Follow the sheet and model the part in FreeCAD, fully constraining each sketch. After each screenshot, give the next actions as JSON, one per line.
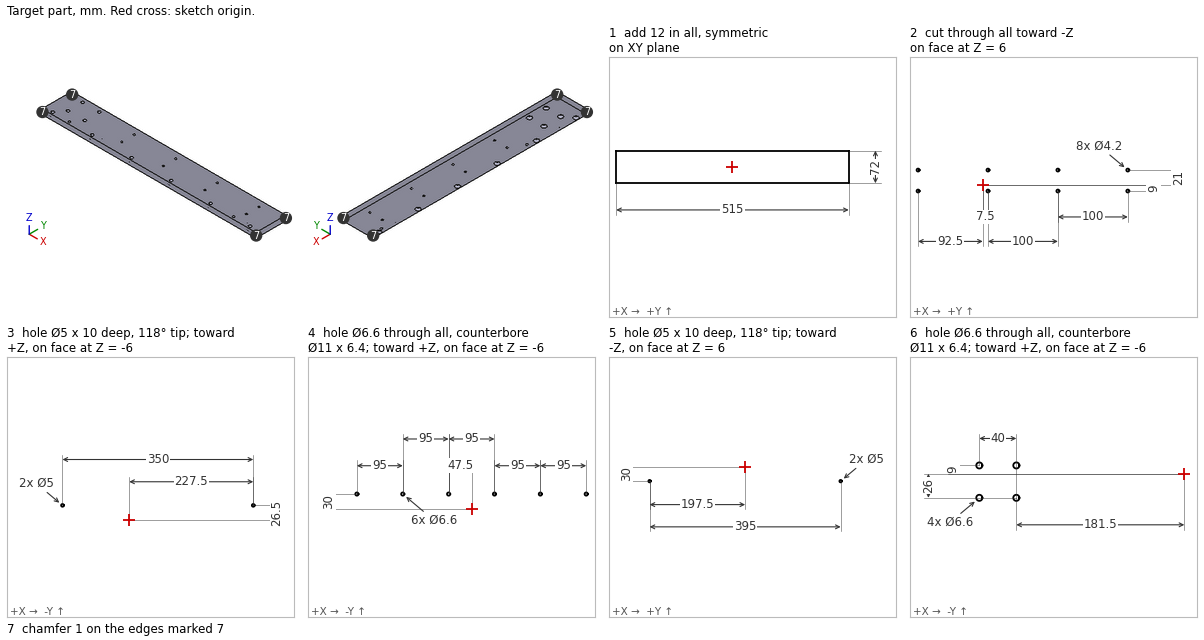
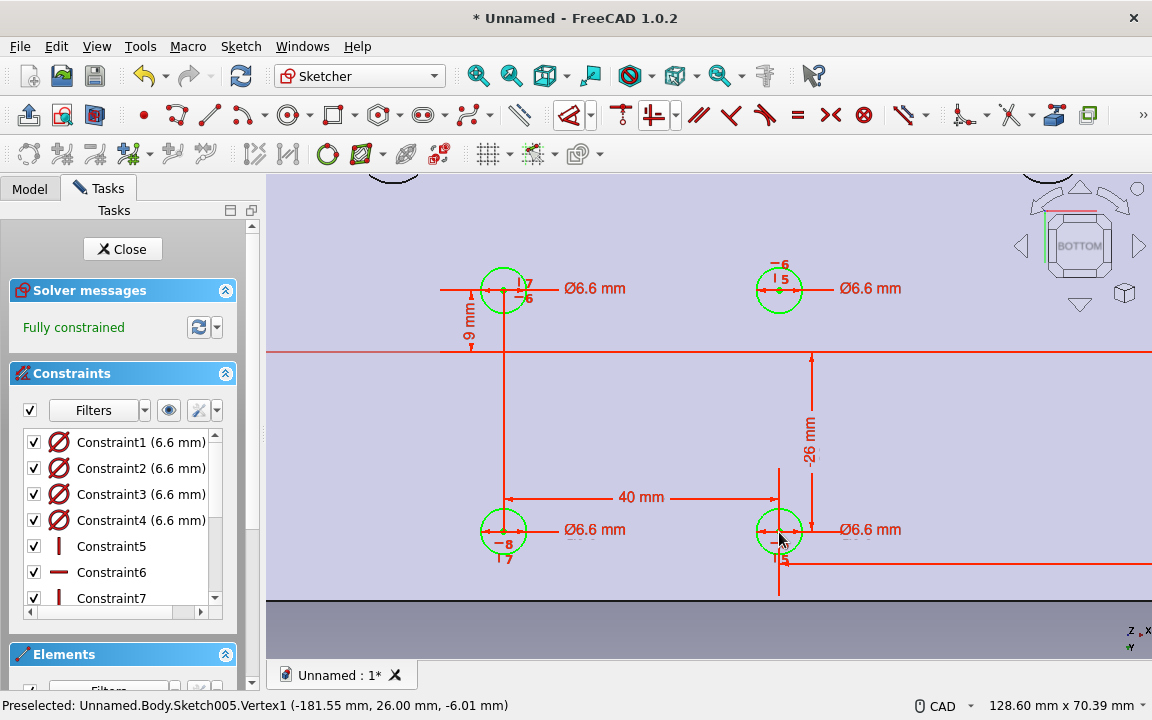
{"action": "left_click", "coordinate": [123, 249]}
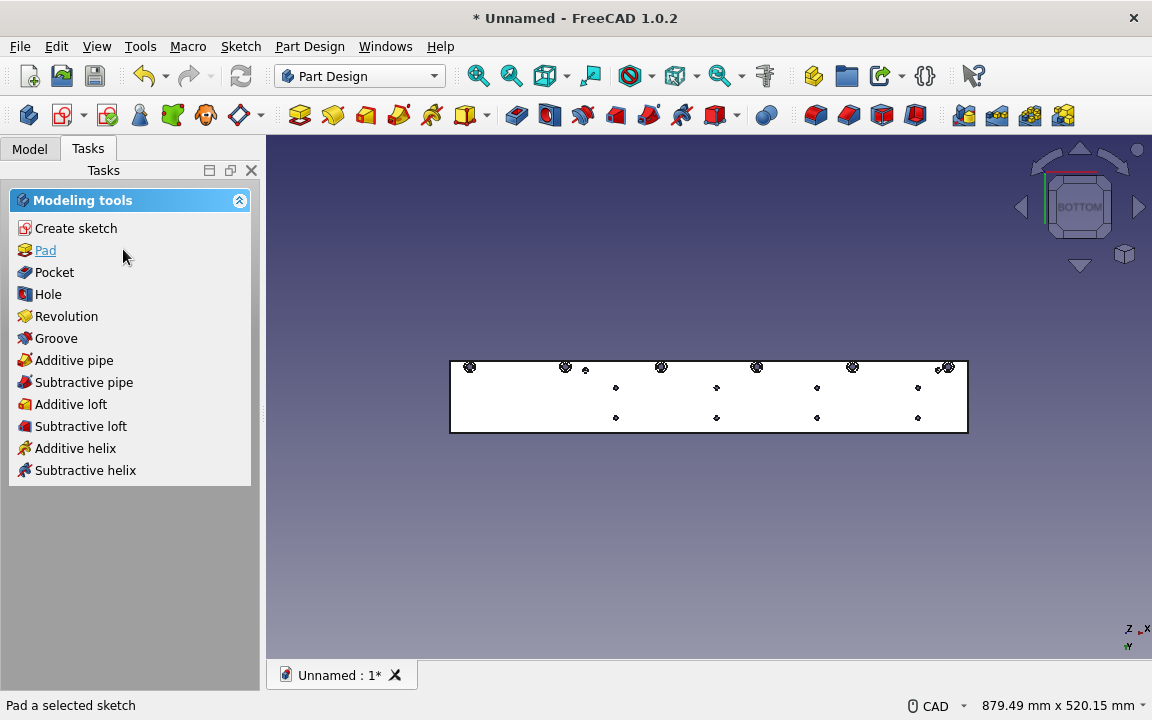
{"action": "left_click", "coordinate": [550, 116]}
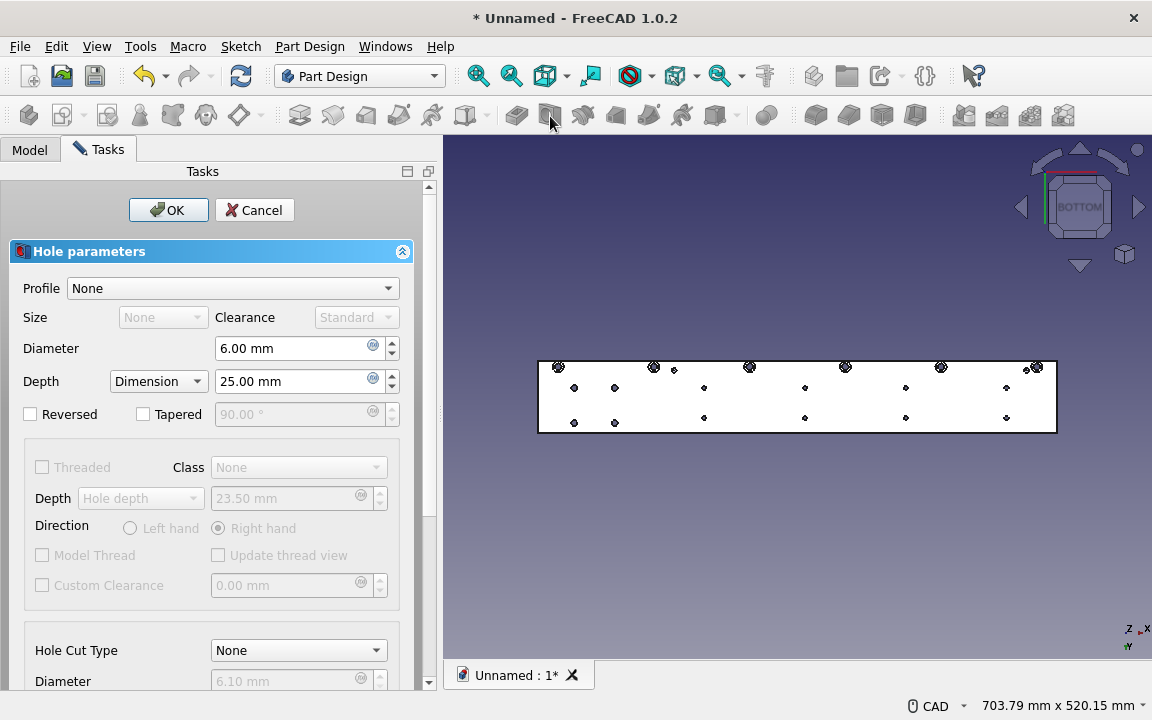
{"action": "triple_click", "coordinate": [300, 348]}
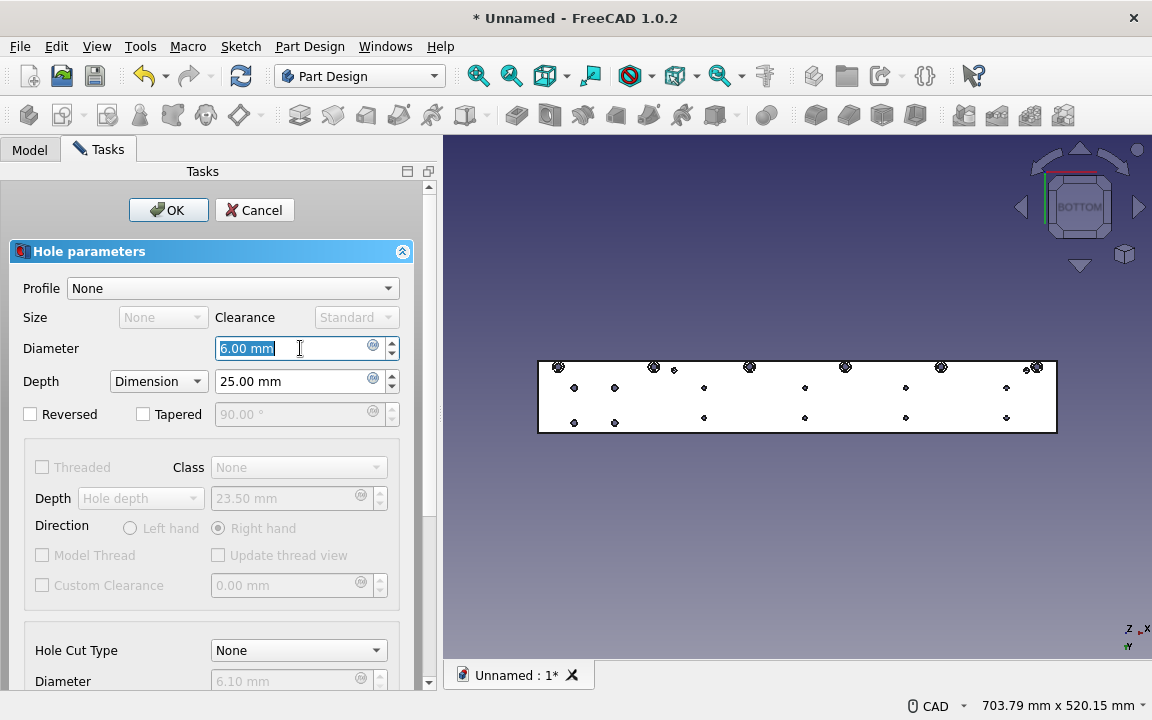
{"action": "type", "text": "6.6"}
{"action": "key", "text": "Tab"}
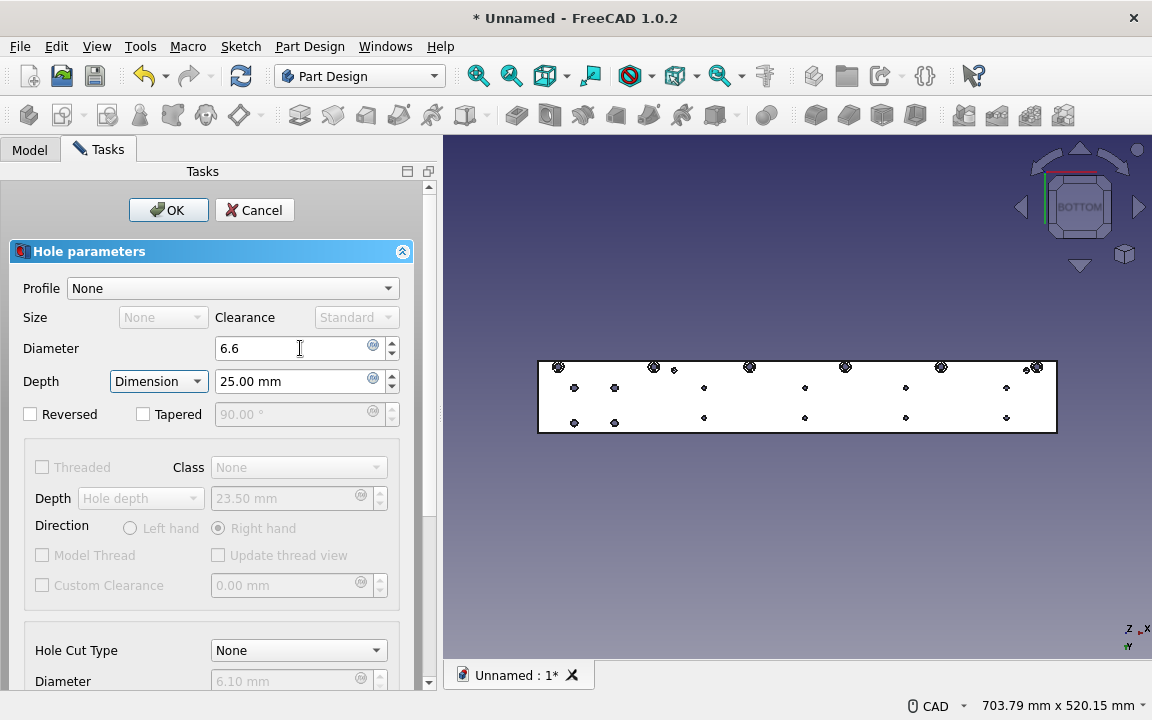
{"action": "left_click", "coordinate": [160, 382]}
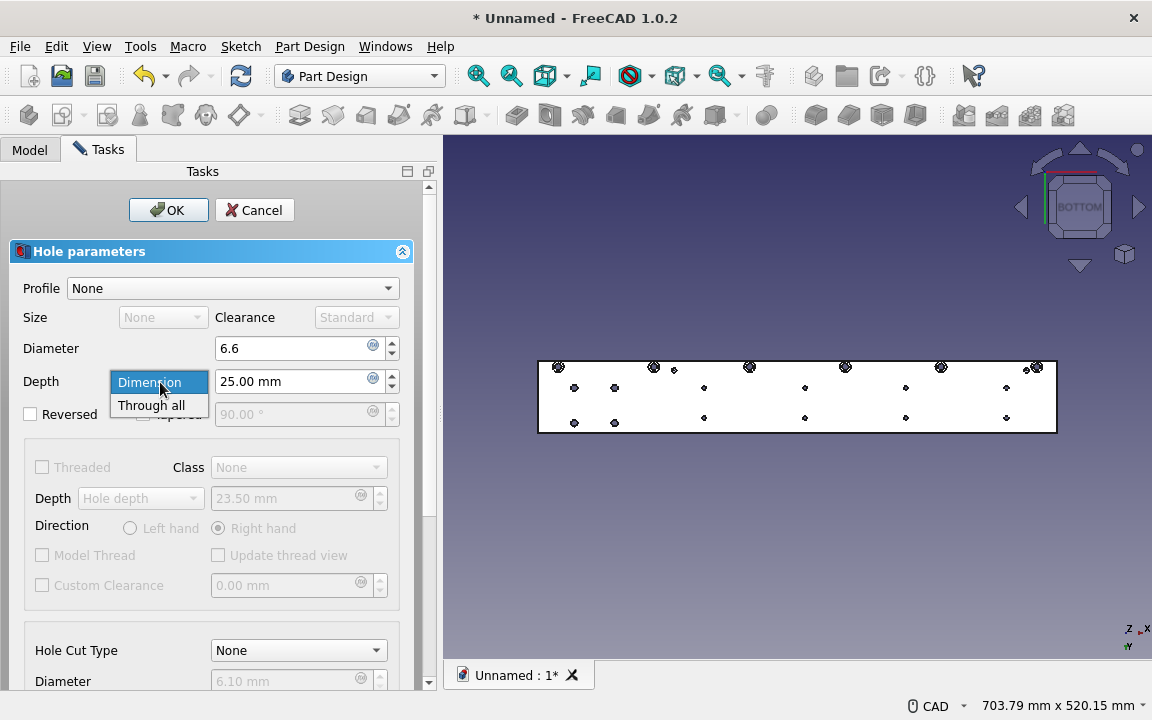
{"action": "left_click", "coordinate": [158, 406]}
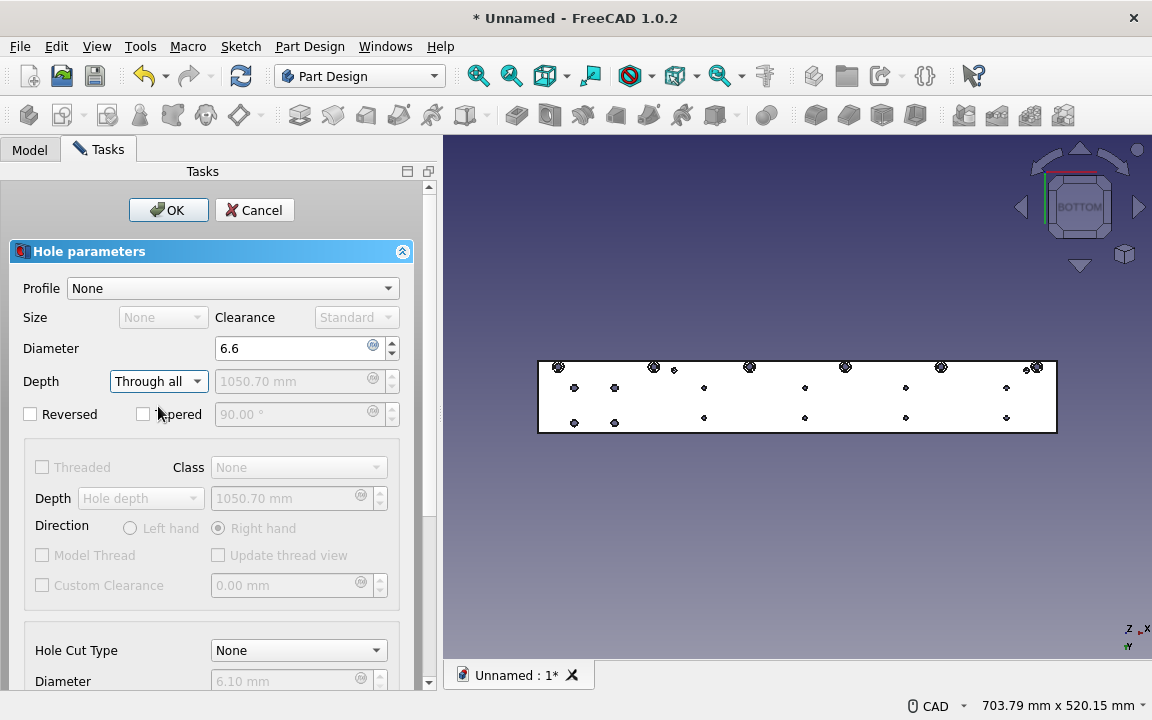
{"action": "left_click", "coordinate": [300, 650]}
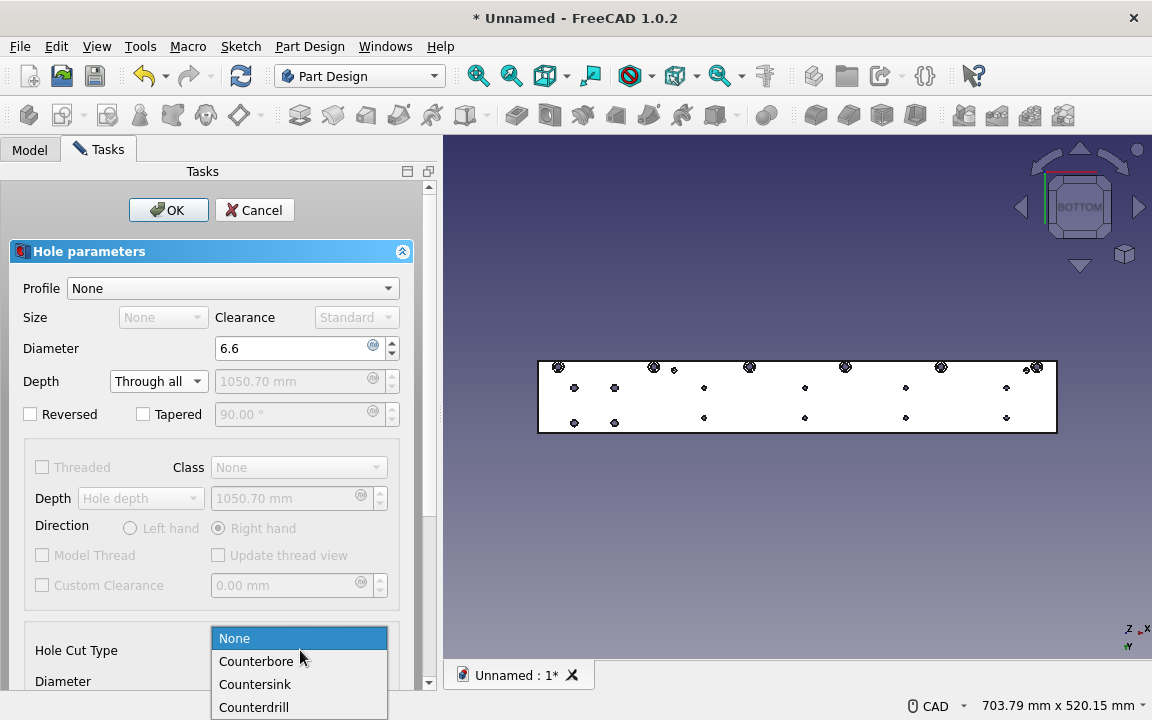
{"action": "left_click", "coordinate": [298, 662]}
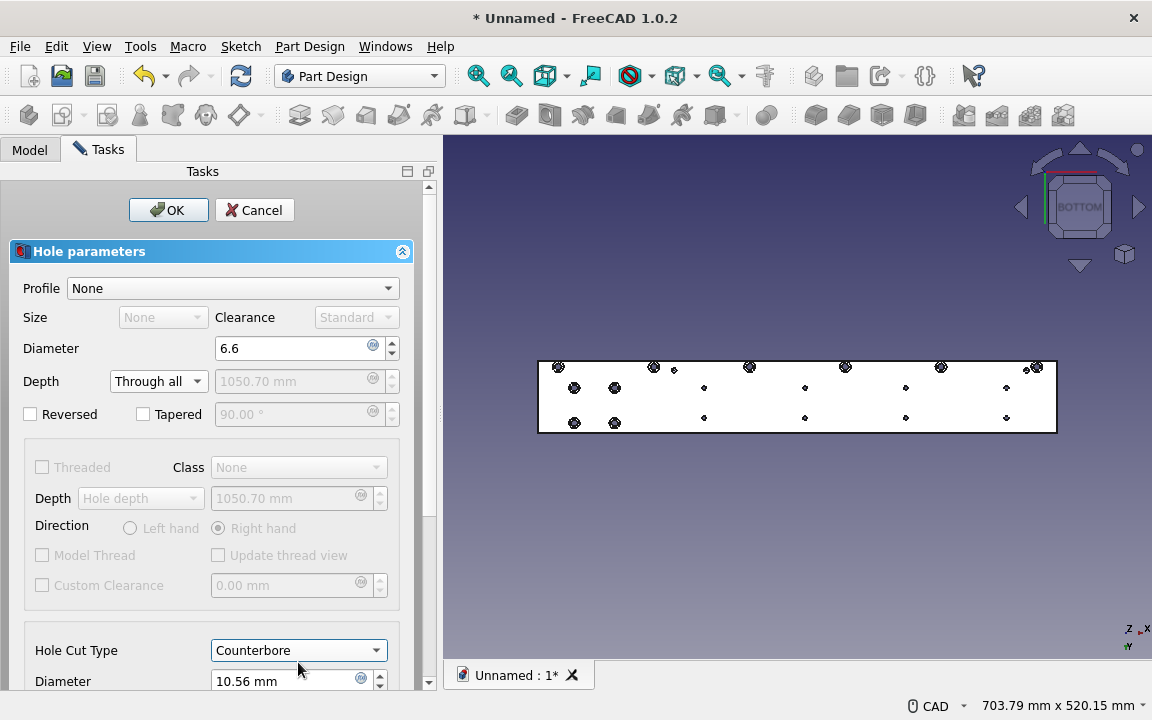
{"action": "scroll", "coordinate": [429, 436], "scroll_direction": "down", "scroll_amount": 2}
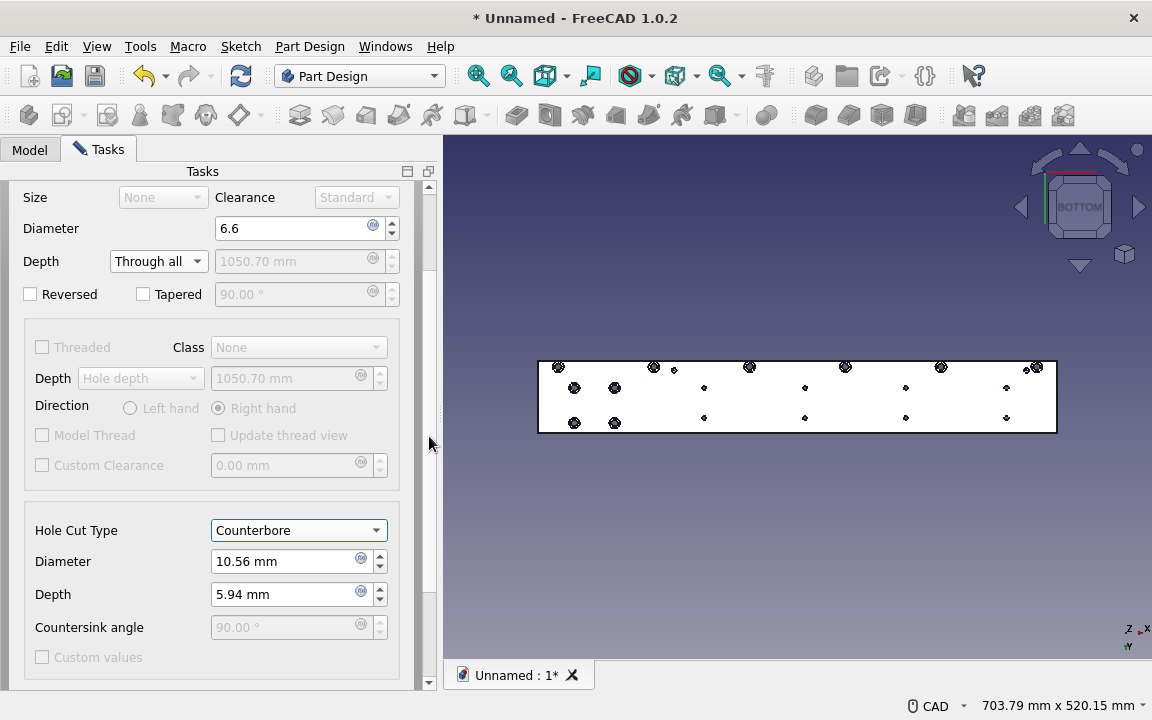
{"action": "triple_click", "coordinate": [292, 562]}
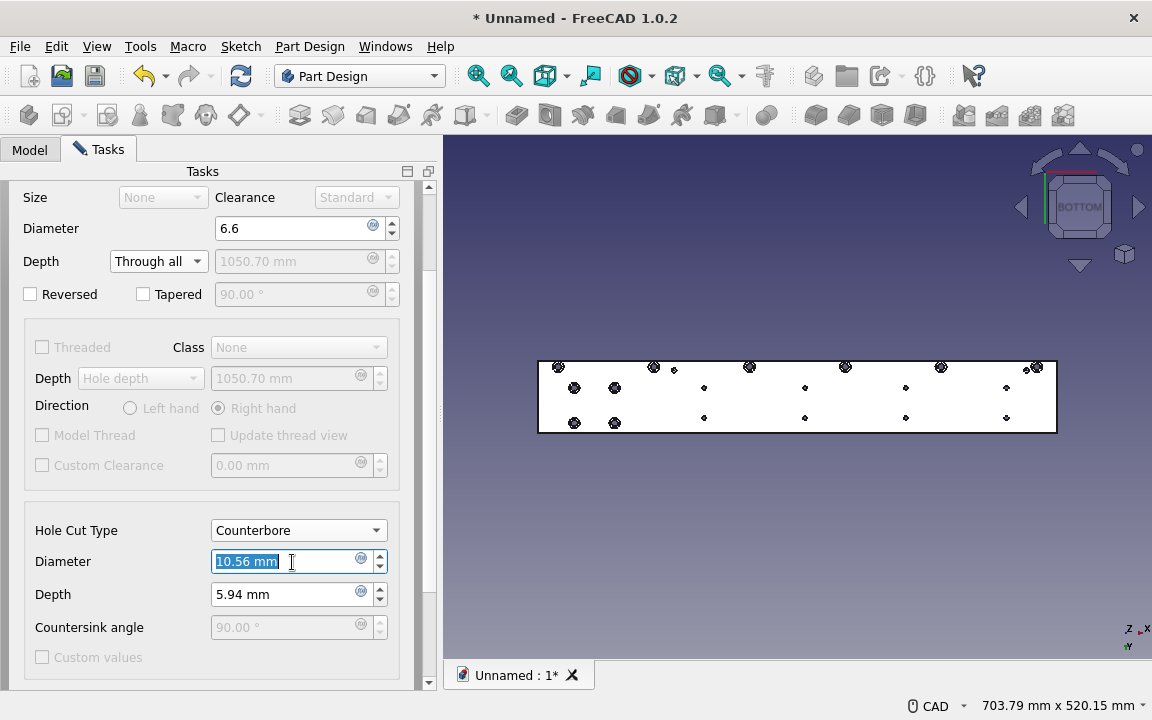
{"action": "type", "text": "11"}
{"action": "key", "text": "Tab"}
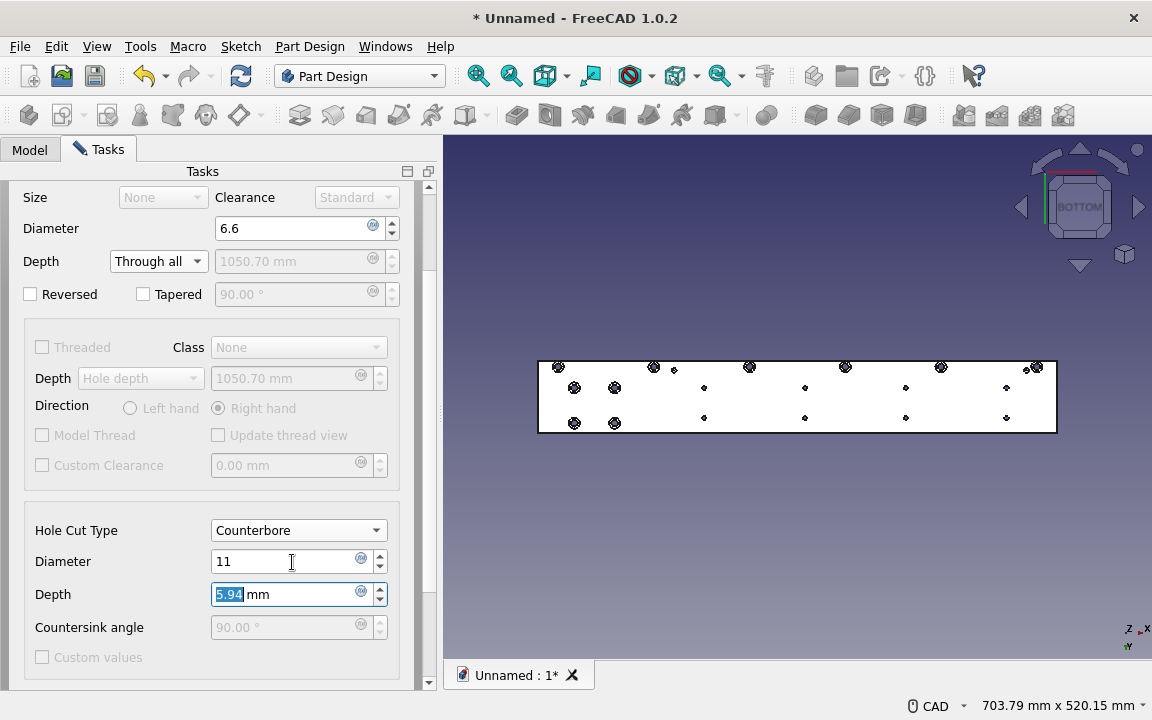
{"action": "type", "text": "6.4"}
{"action": "key", "text": "Tab"}